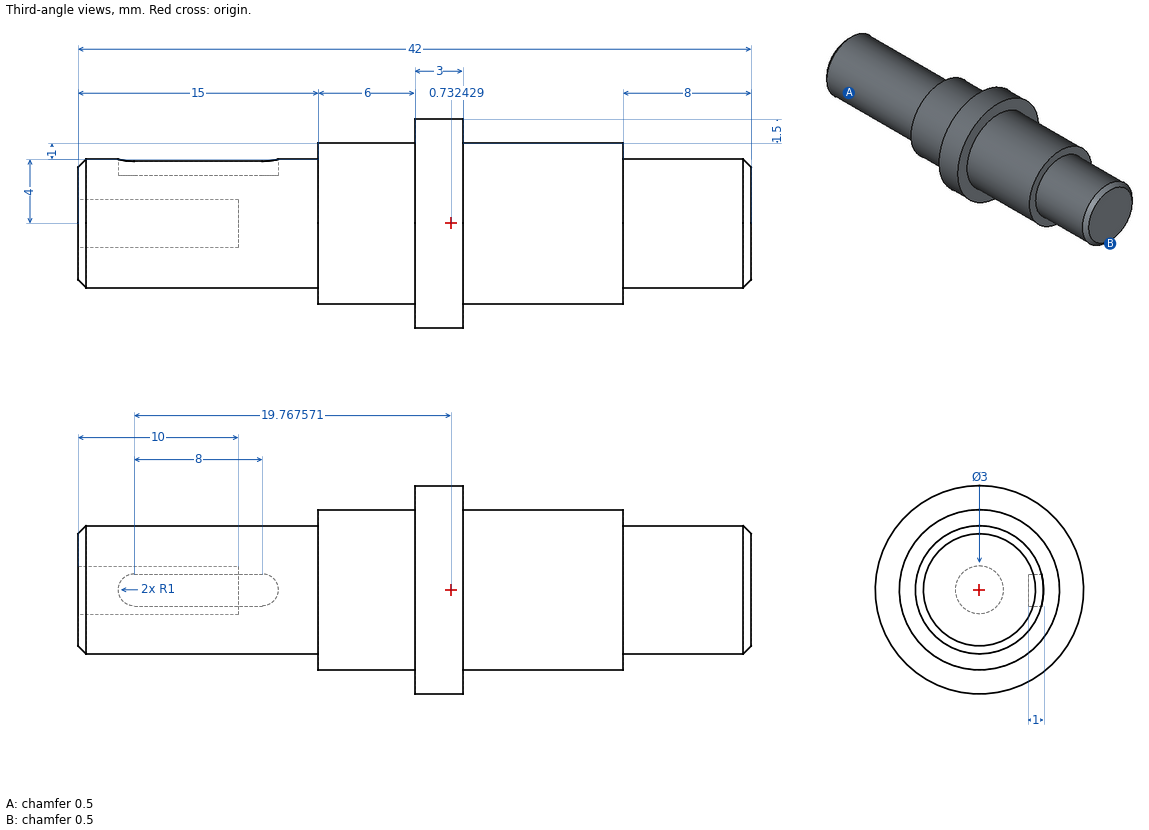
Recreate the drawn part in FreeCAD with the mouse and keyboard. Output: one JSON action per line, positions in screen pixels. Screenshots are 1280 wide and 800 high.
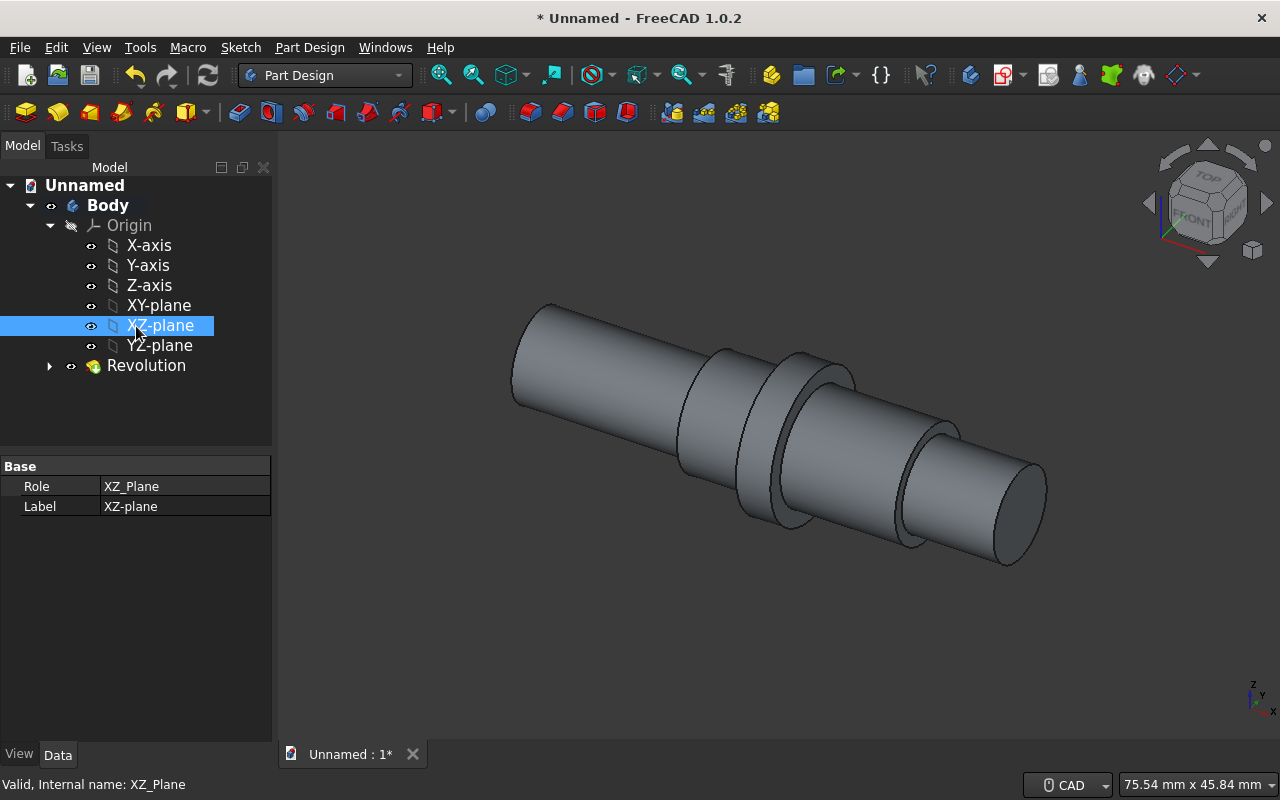
{"action": "left_click", "coordinate": [1176, 76]}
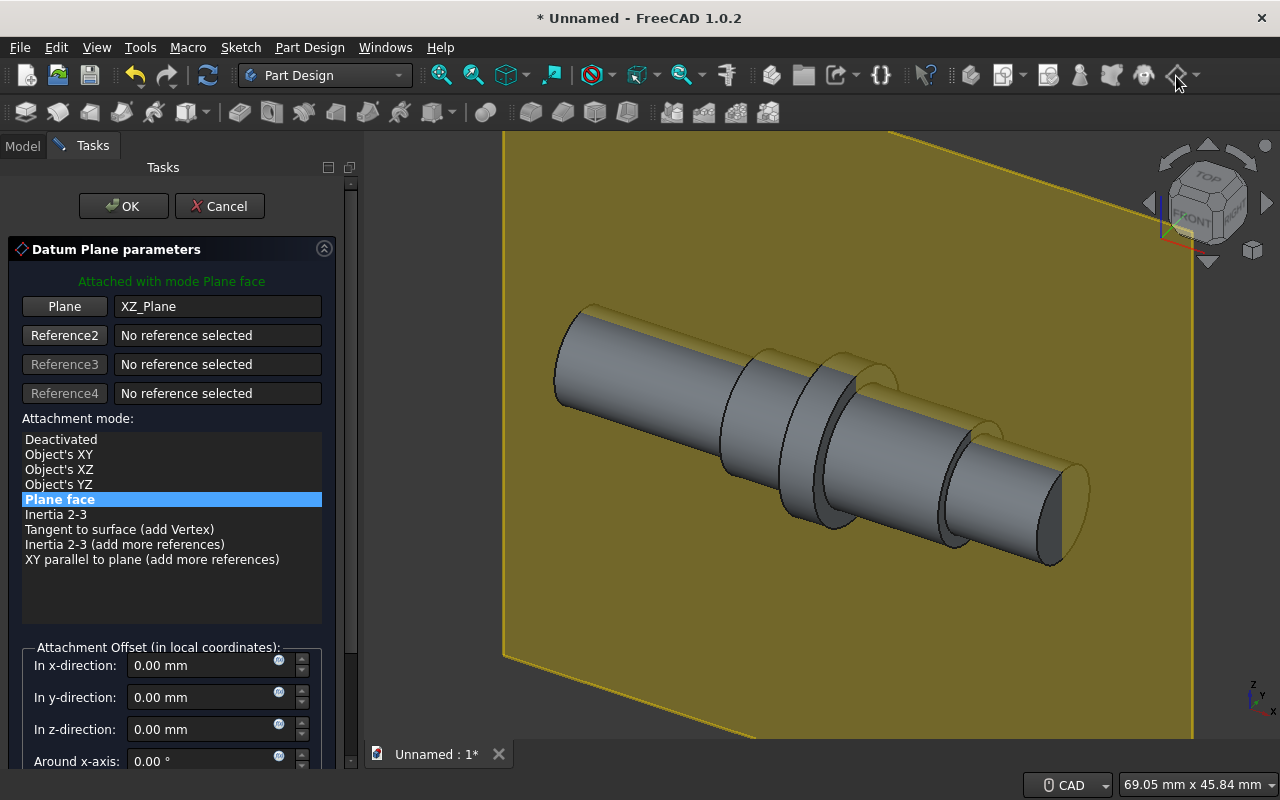
{"action": "triple_click", "coordinate": [210, 729]}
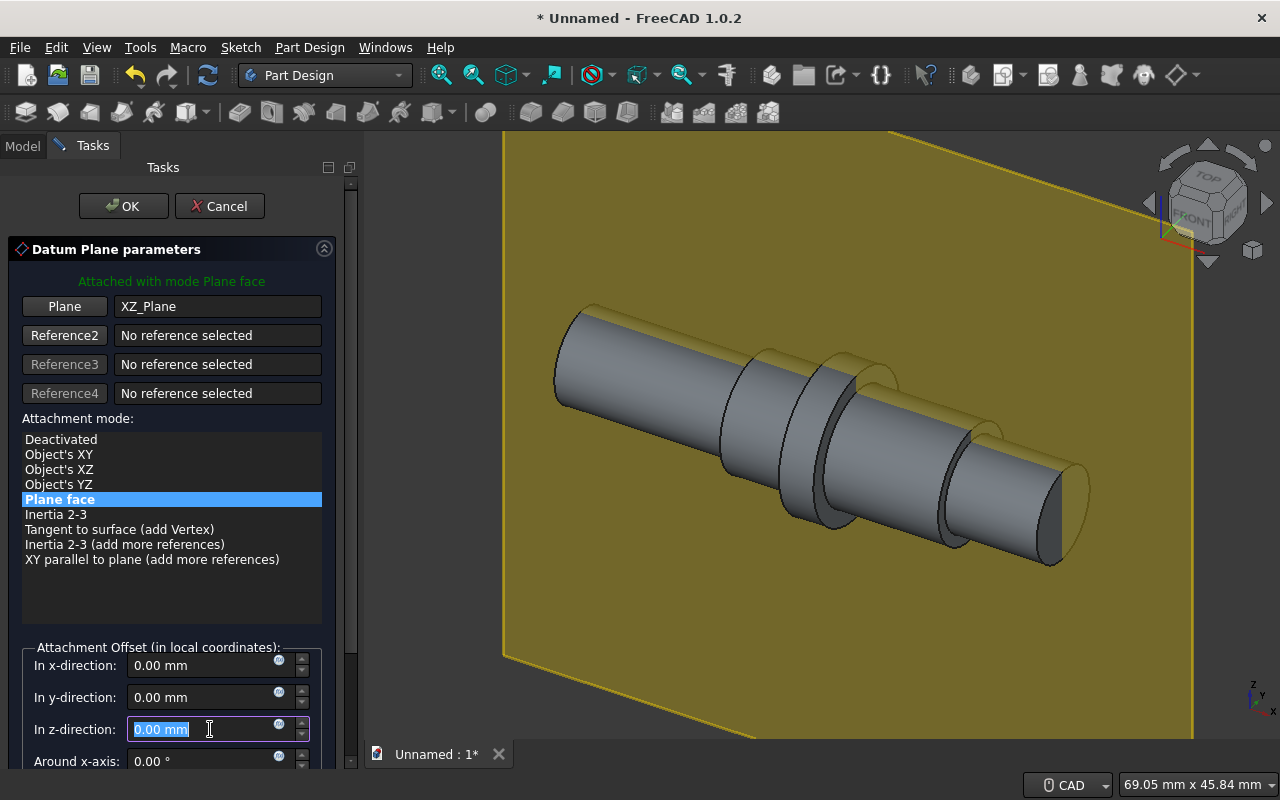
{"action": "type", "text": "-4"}
{"action": "key", "text": "Tab"}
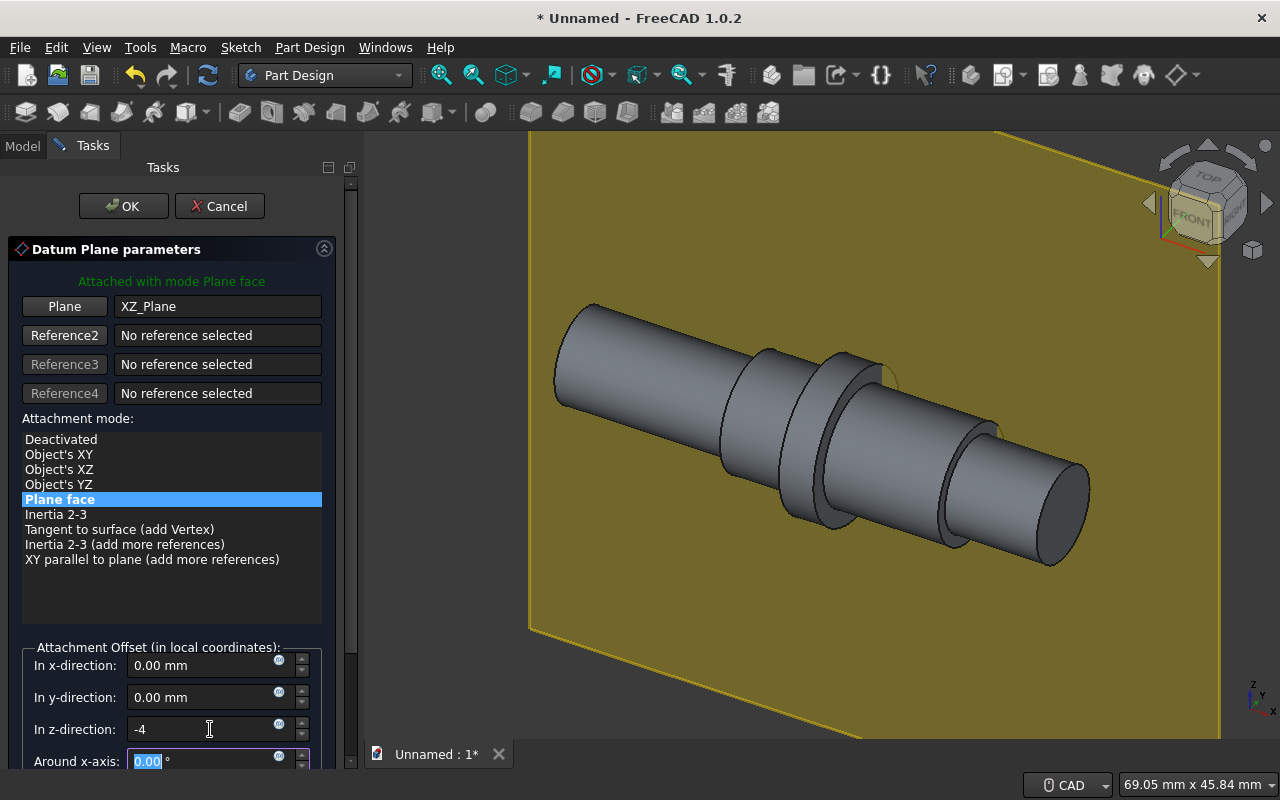
{"action": "left_click", "coordinate": [124, 206]}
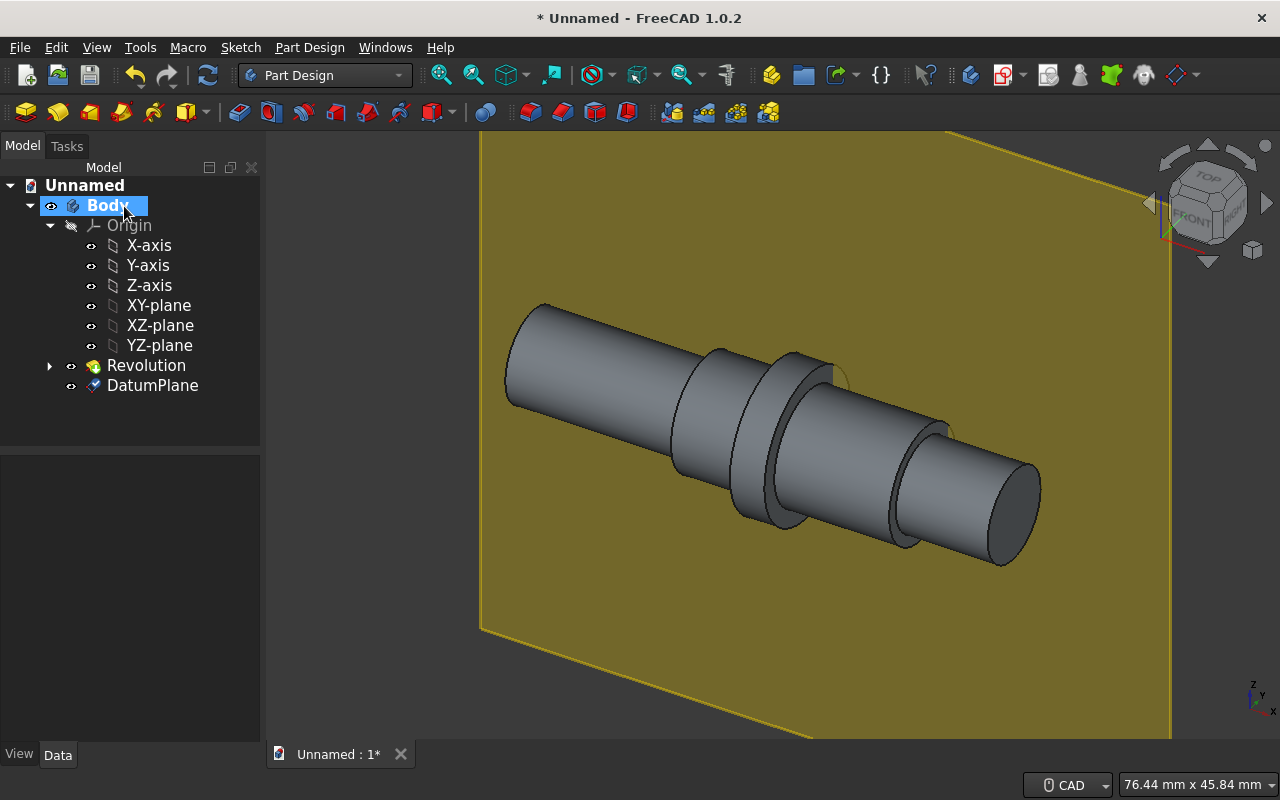
{"action": "left_click", "coordinate": [116, 386]}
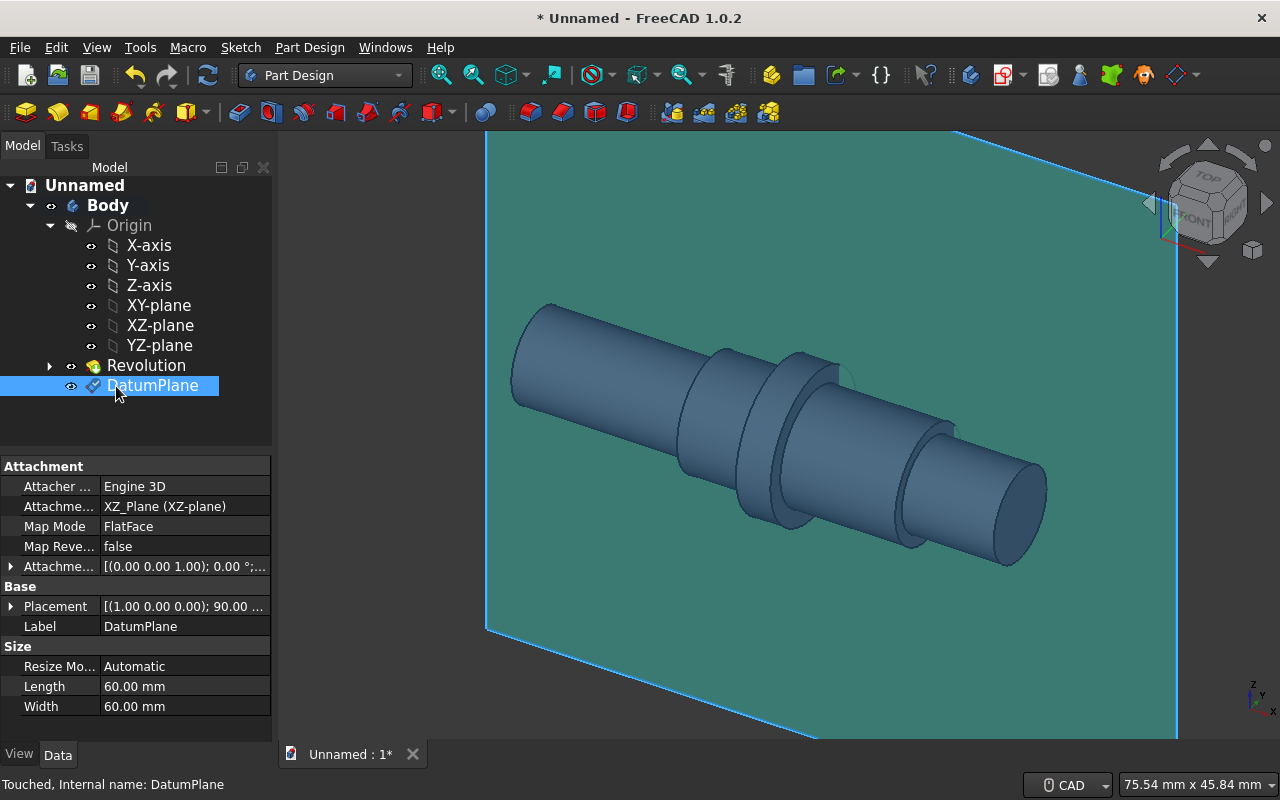
{"action": "left_click", "coordinate": [1004, 76]}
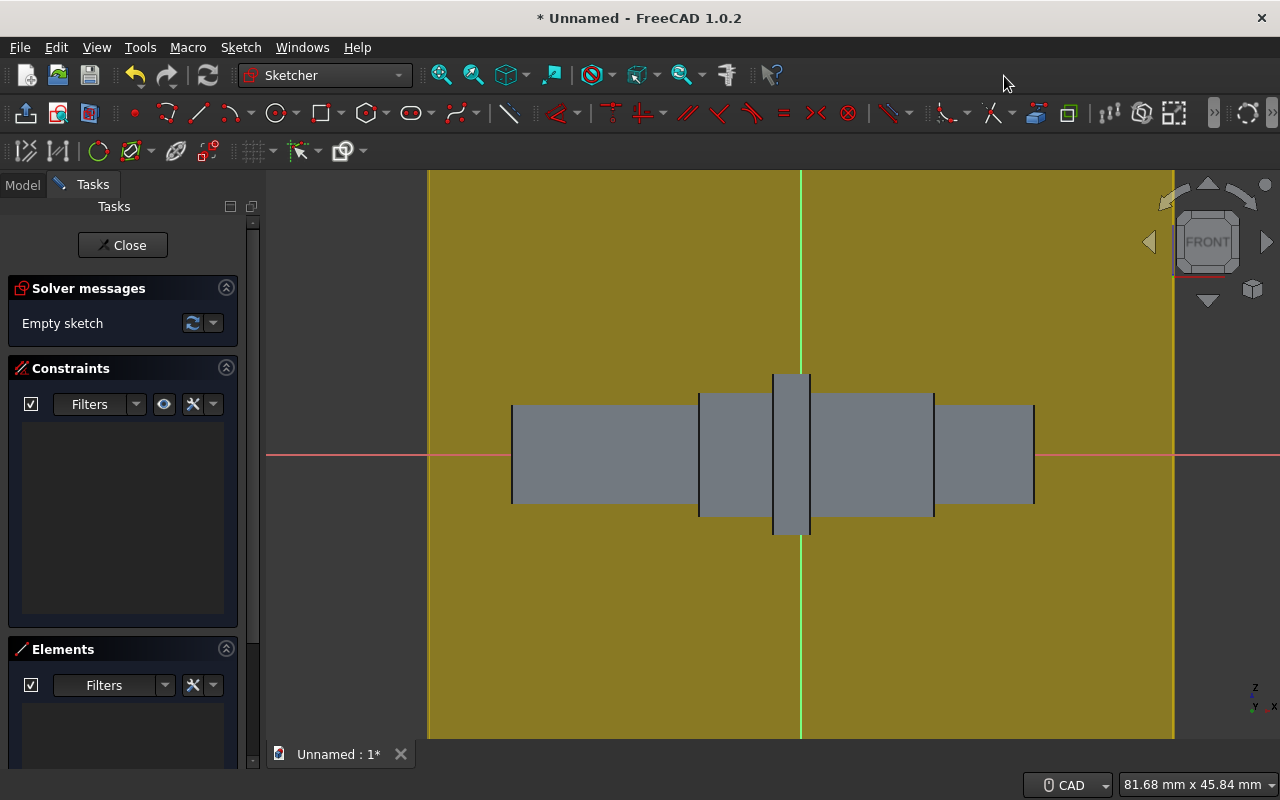
{"action": "left_click", "coordinate": [90, 114]}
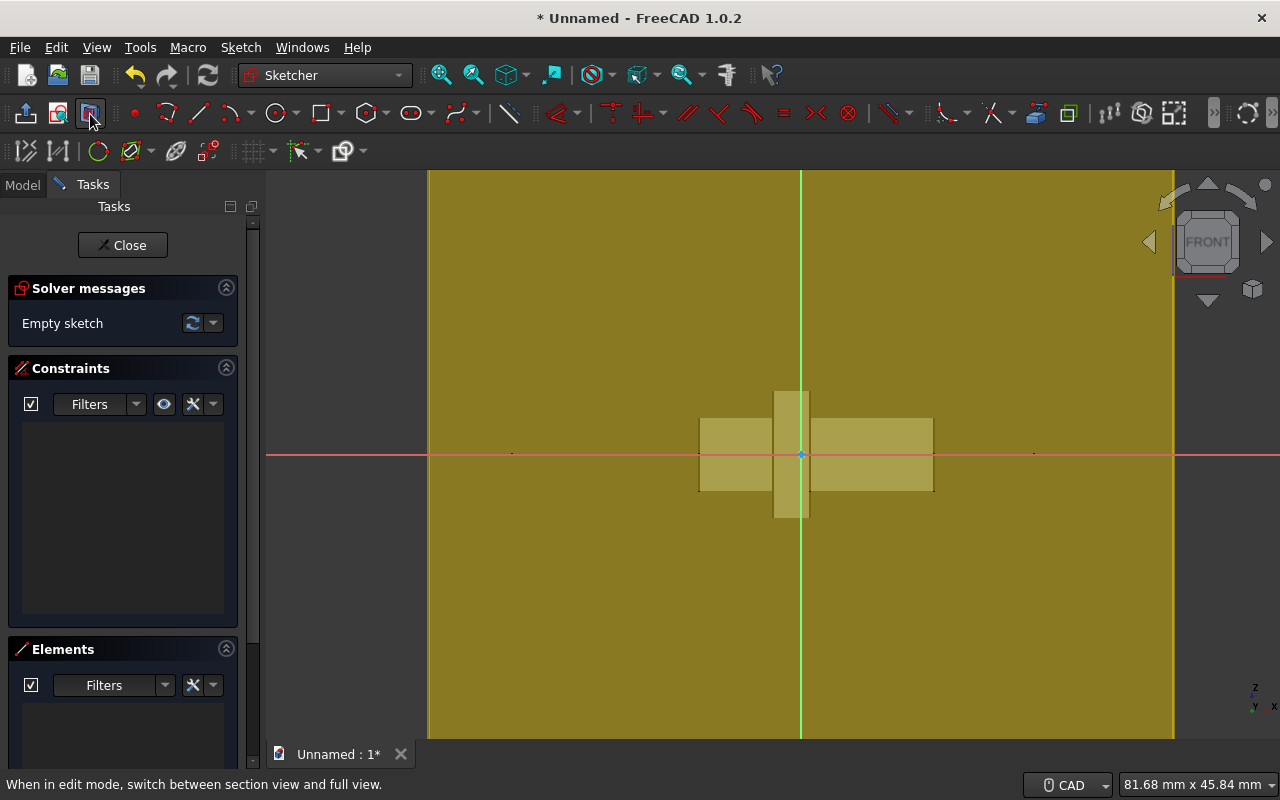
{"action": "scroll", "coordinate": [646, 455], "scroll_direction": "up", "scroll_amount": 4}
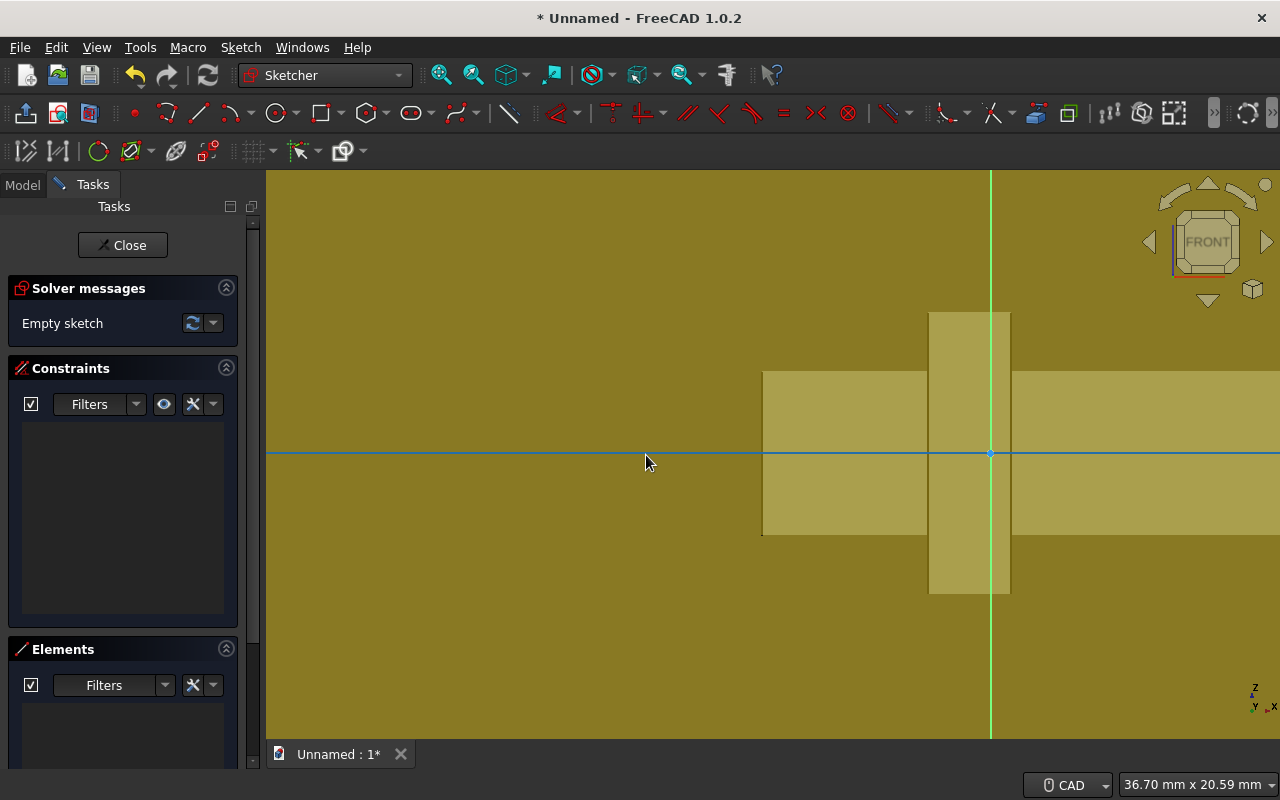
{"action": "left_click", "coordinate": [412, 114]}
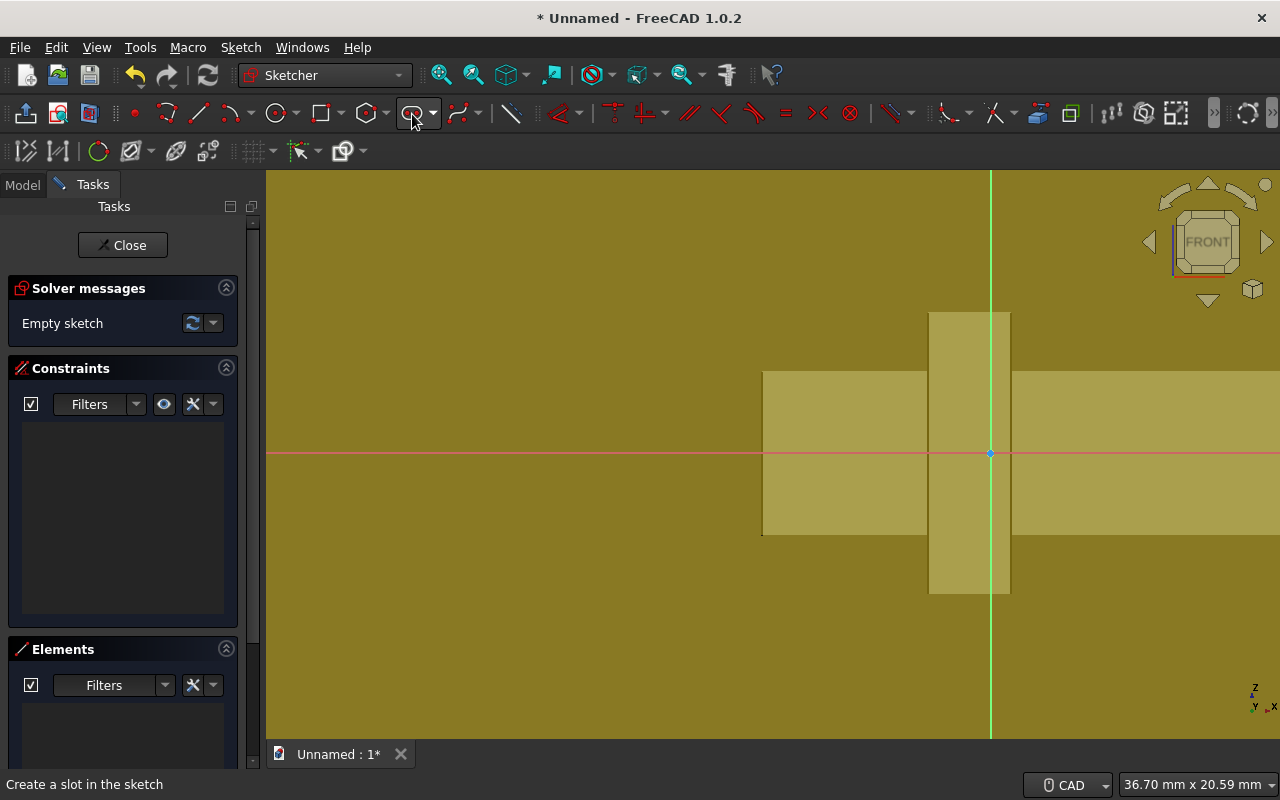
{"action": "left_click", "coordinate": [445, 453]}